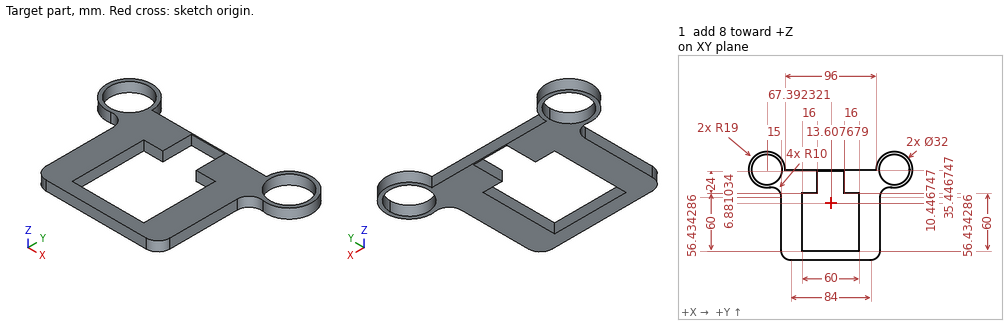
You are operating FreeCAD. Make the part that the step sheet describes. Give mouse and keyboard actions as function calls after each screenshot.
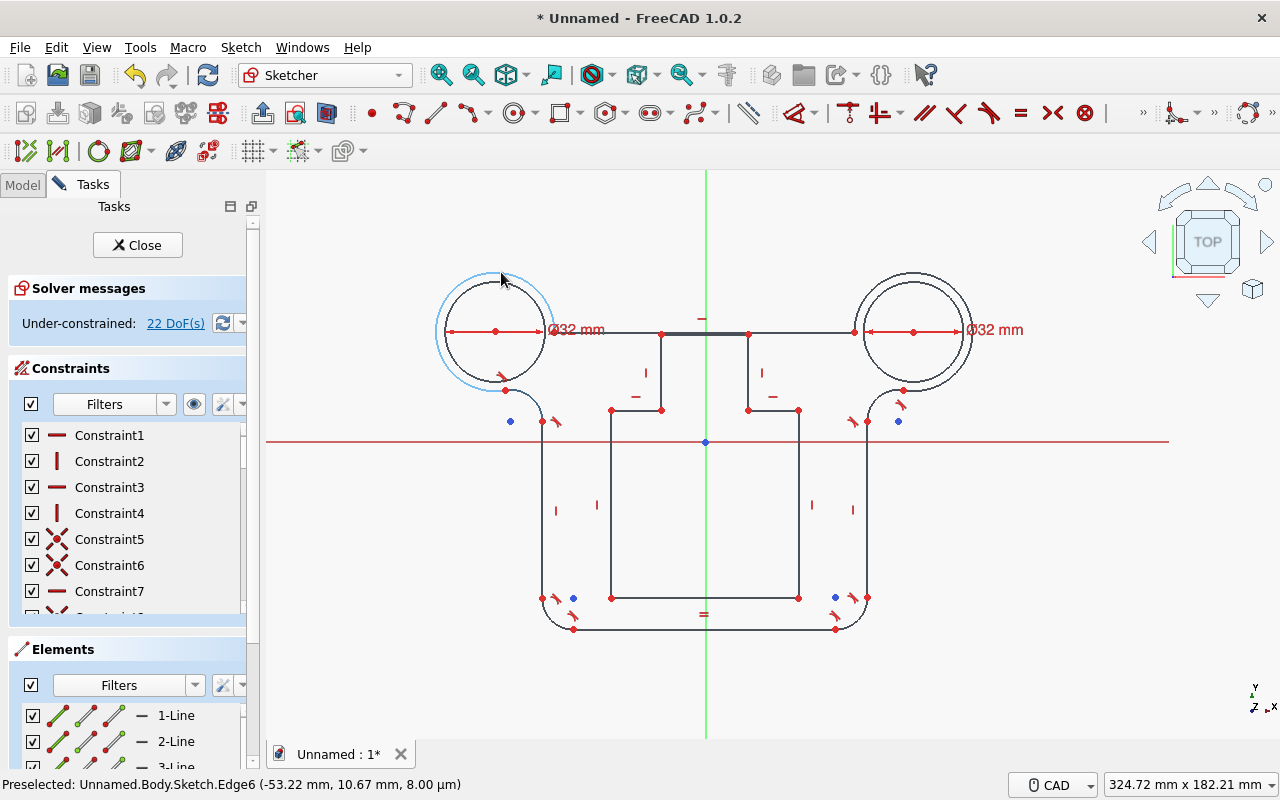
click(546, 613)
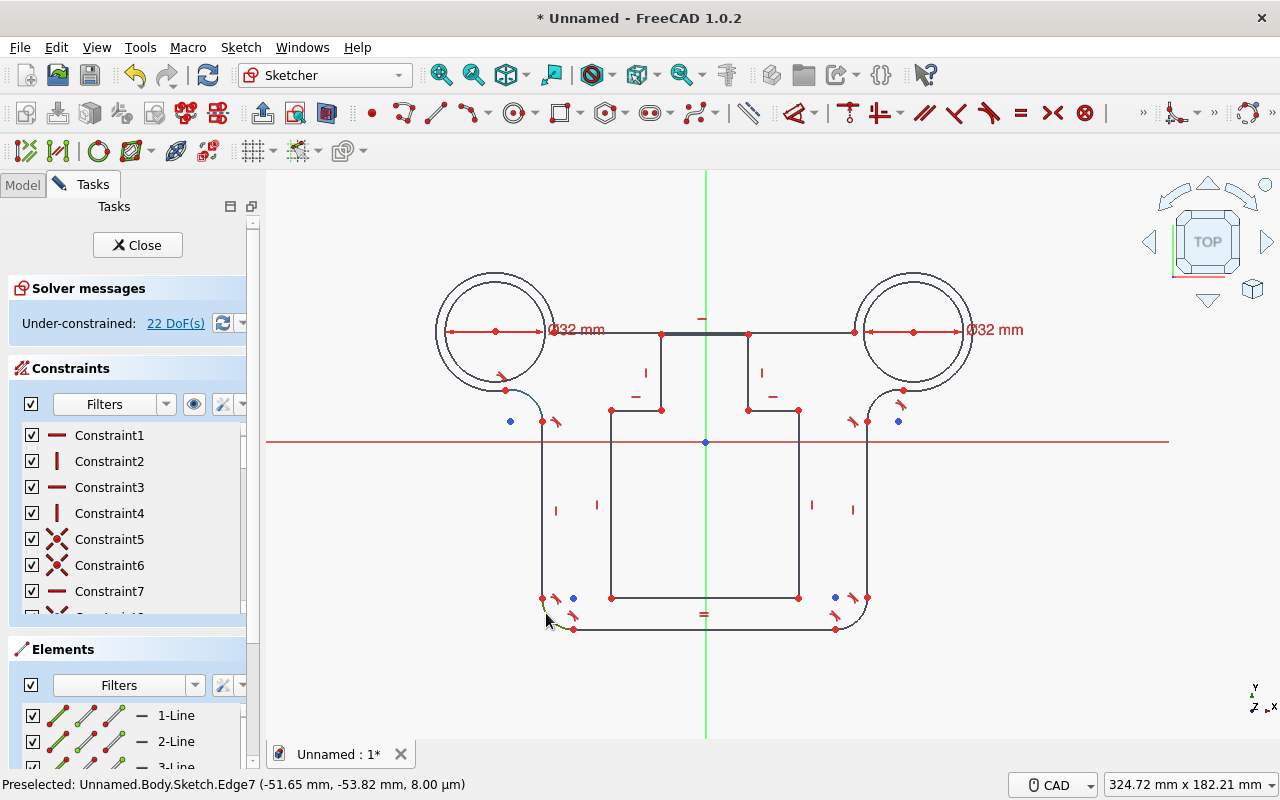
click(850, 626)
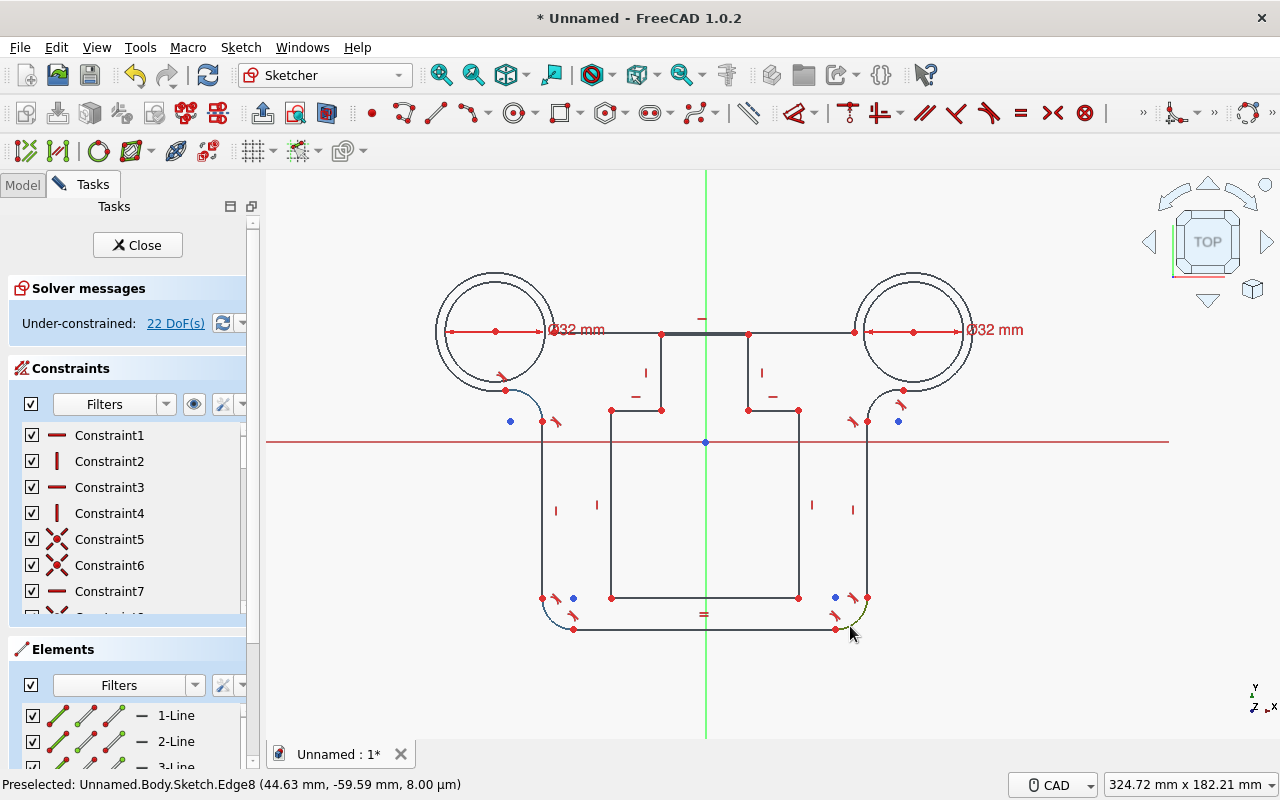
click(888, 392)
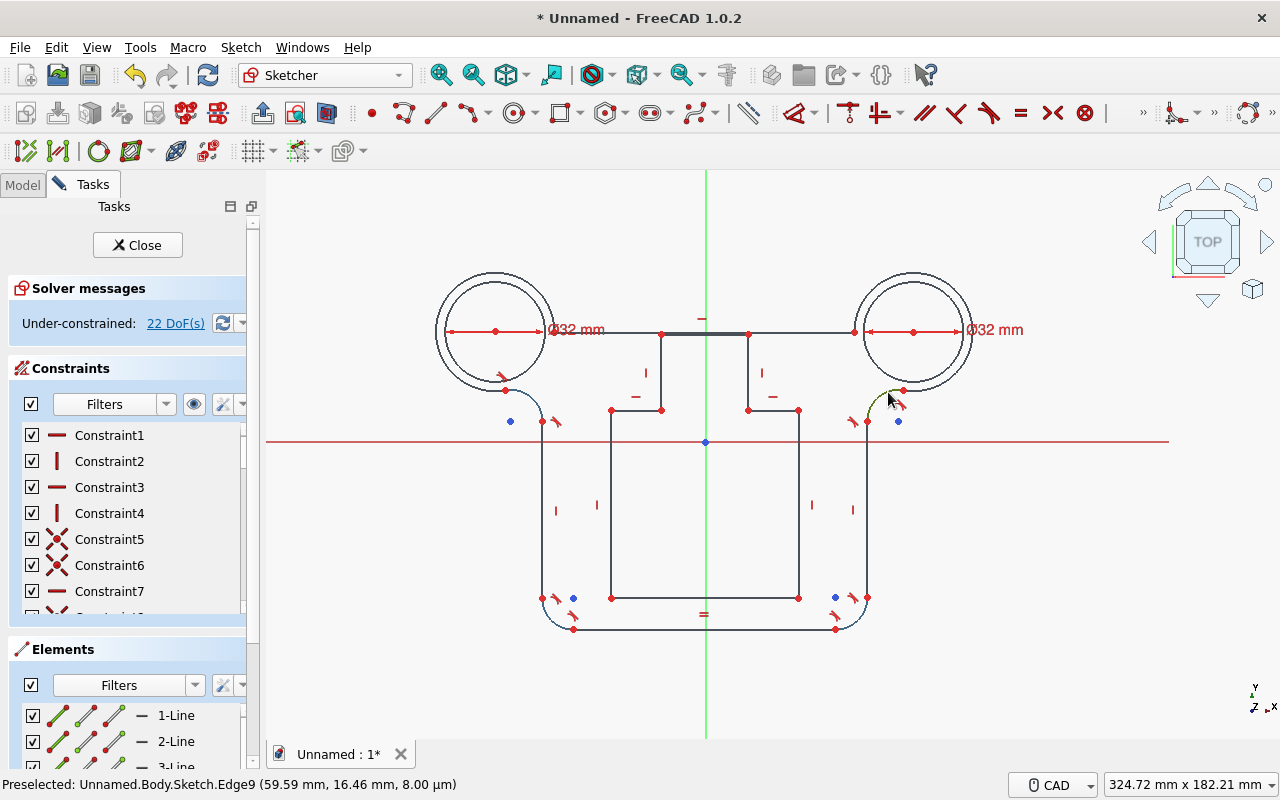
click(1022, 114)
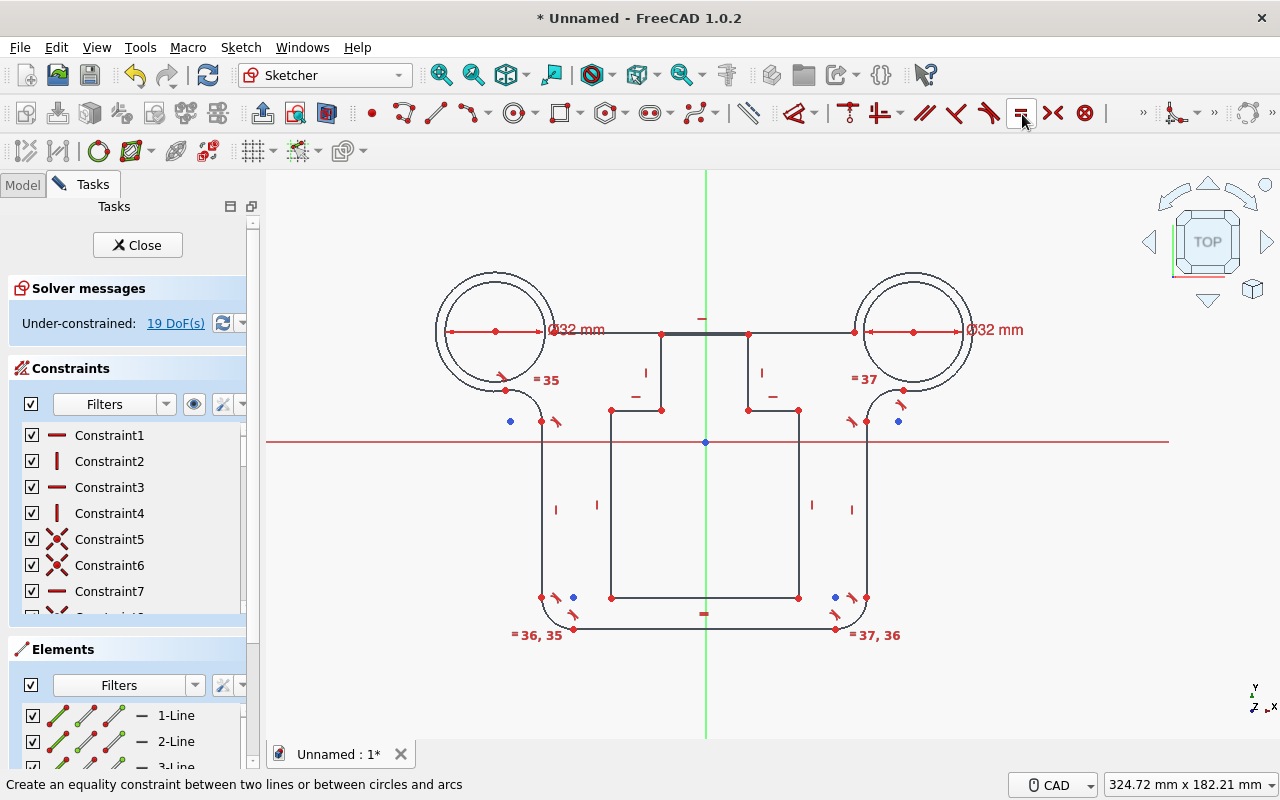
scroll(502, 273, up, 2)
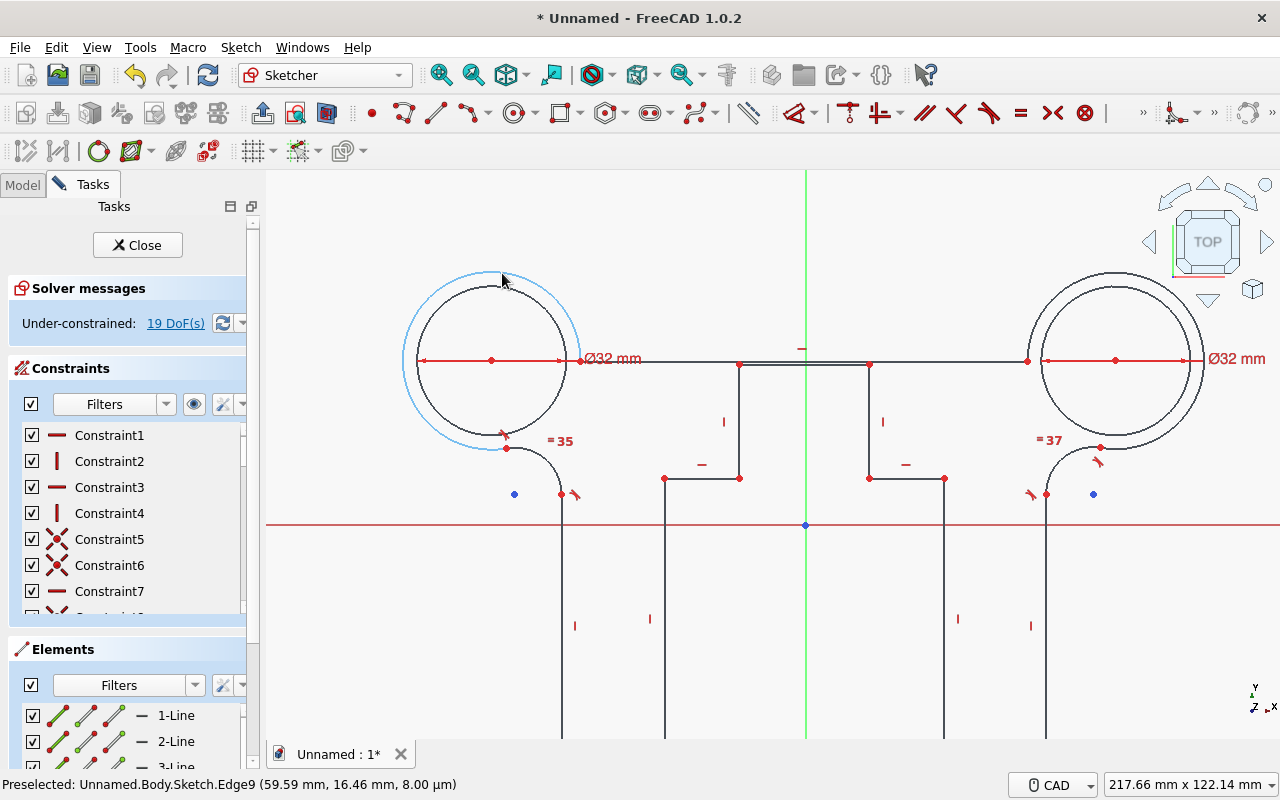
click(502, 273)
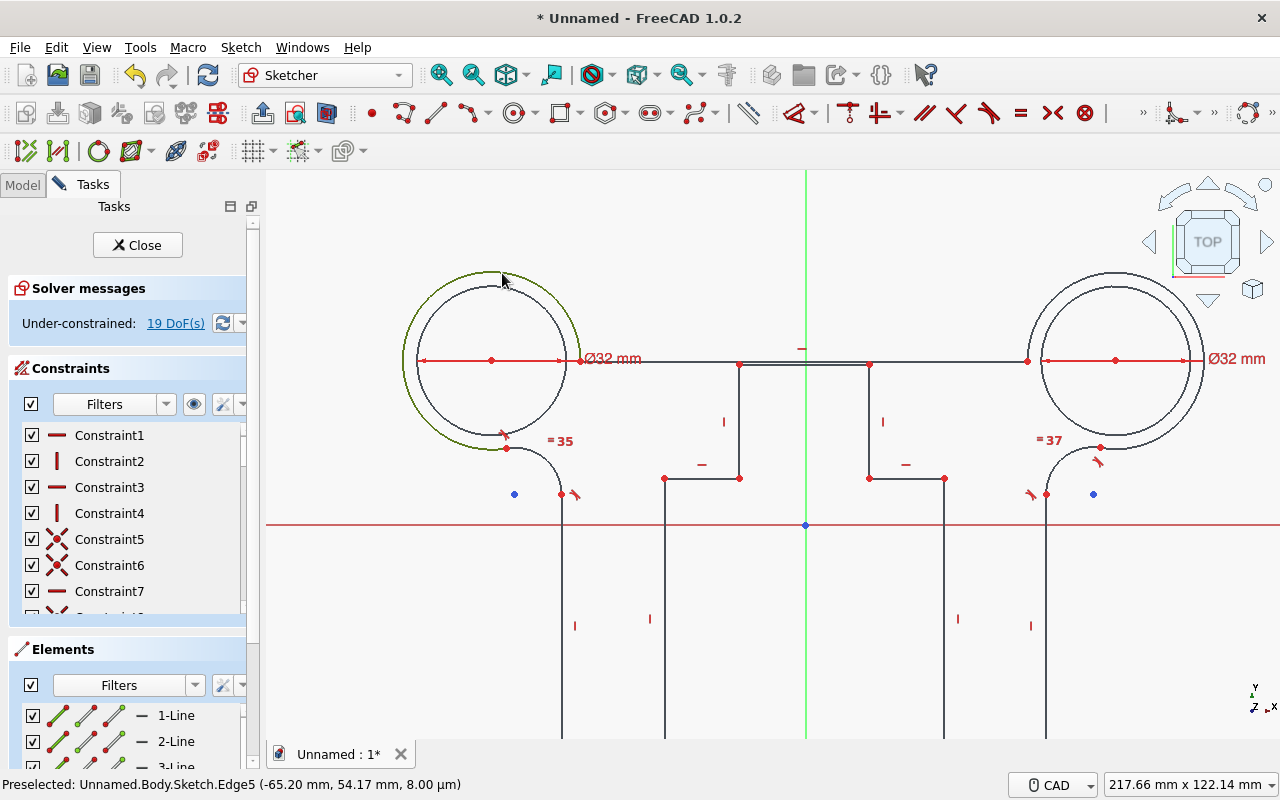
click(1106, 273)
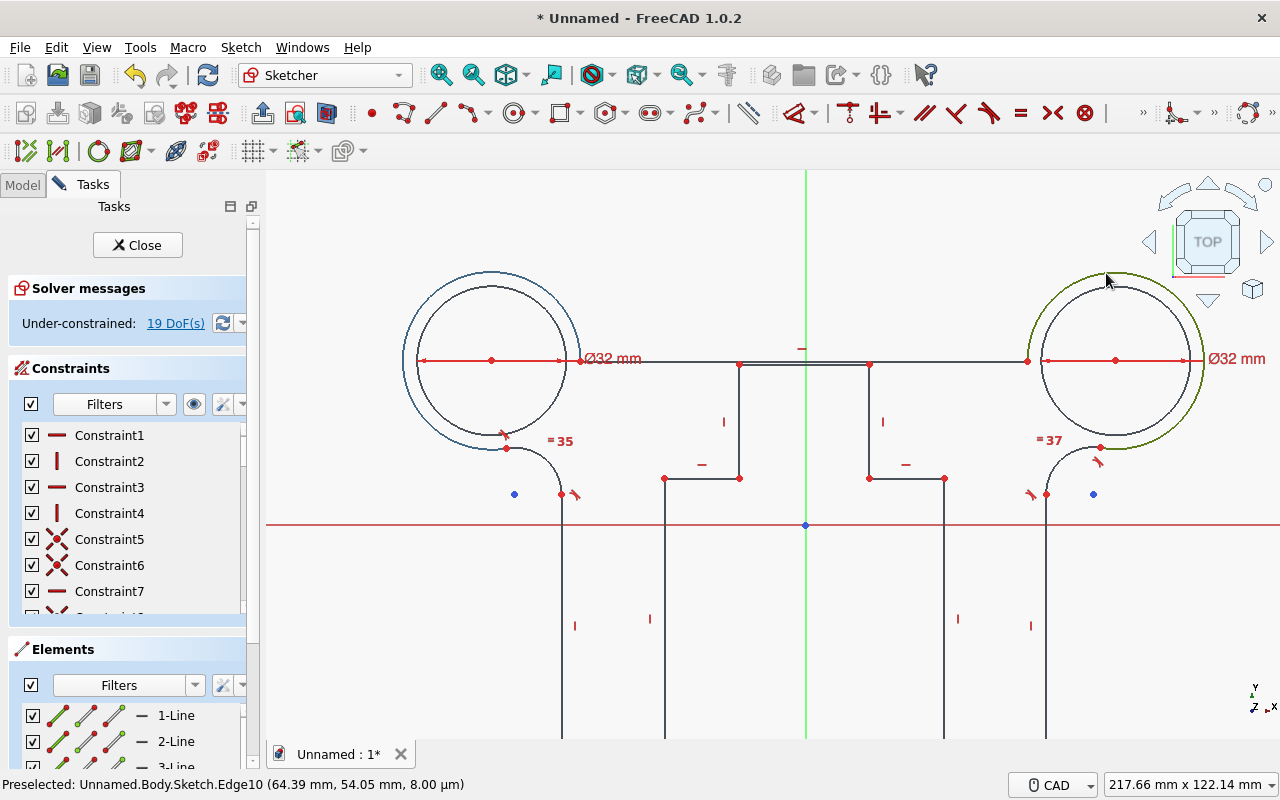
click(1022, 114)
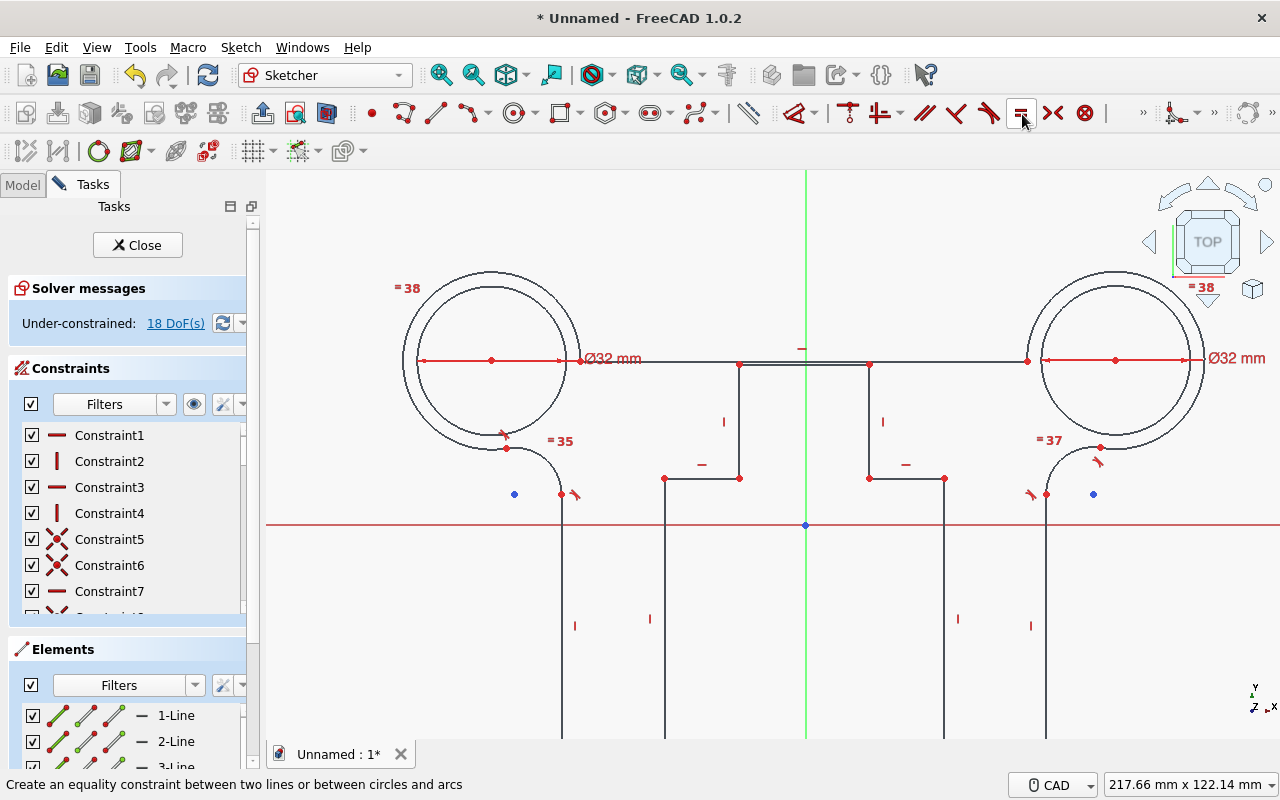
click(794, 114)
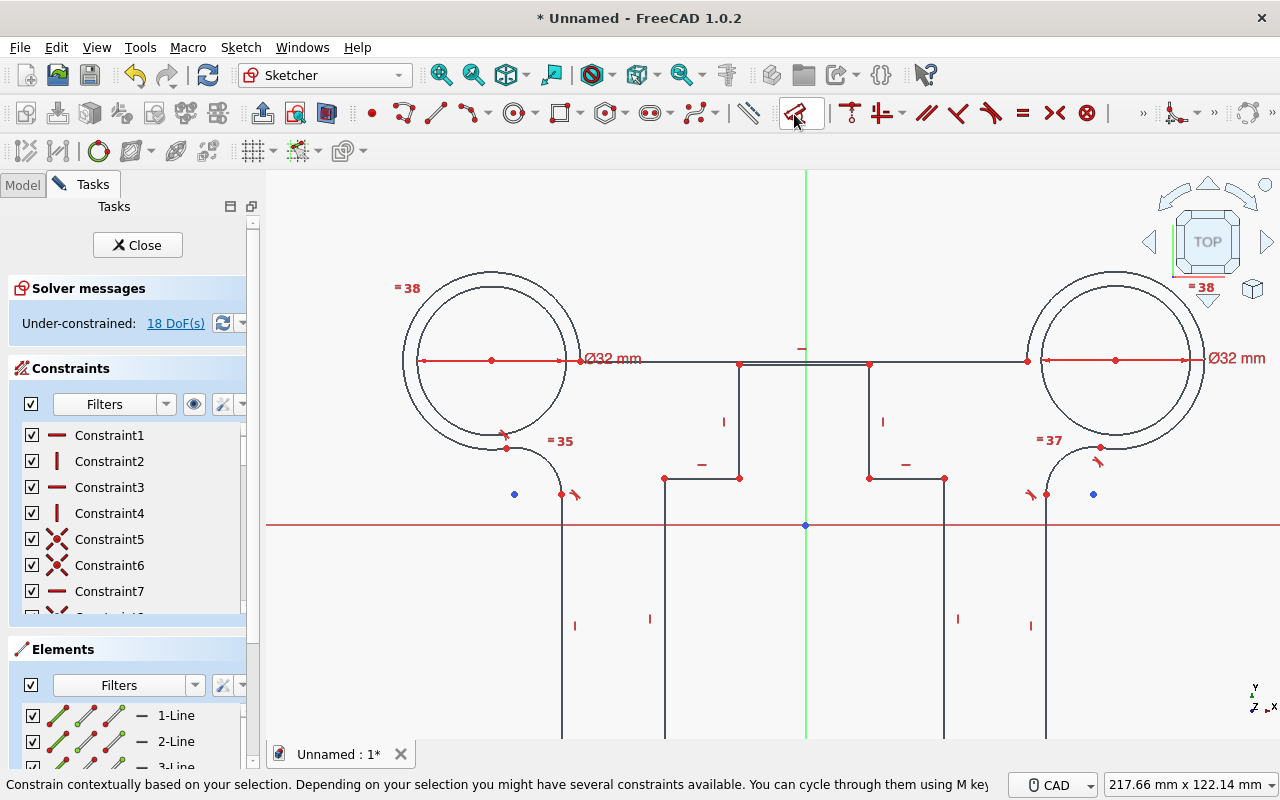
click(502, 273)
click(506, 241)